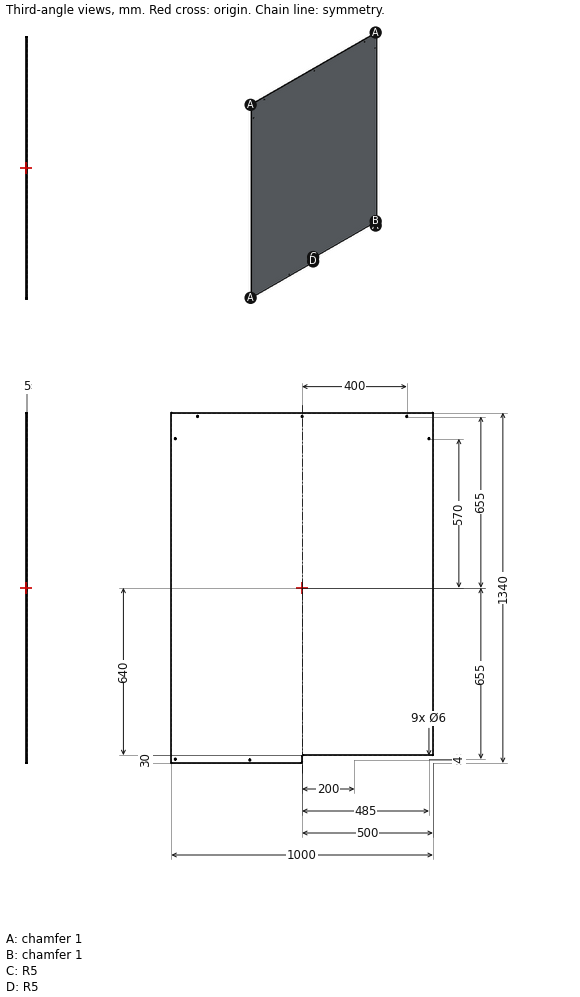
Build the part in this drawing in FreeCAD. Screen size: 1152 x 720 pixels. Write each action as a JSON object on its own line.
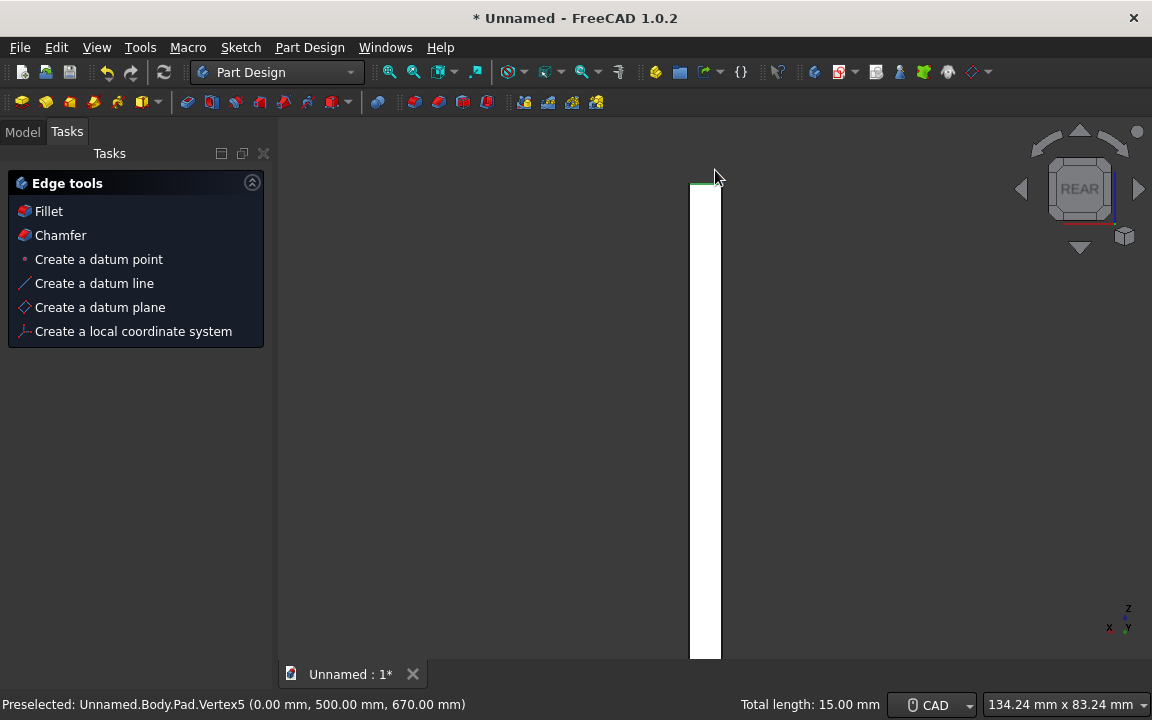
{"action": "left_click", "coordinate": [390, 72]}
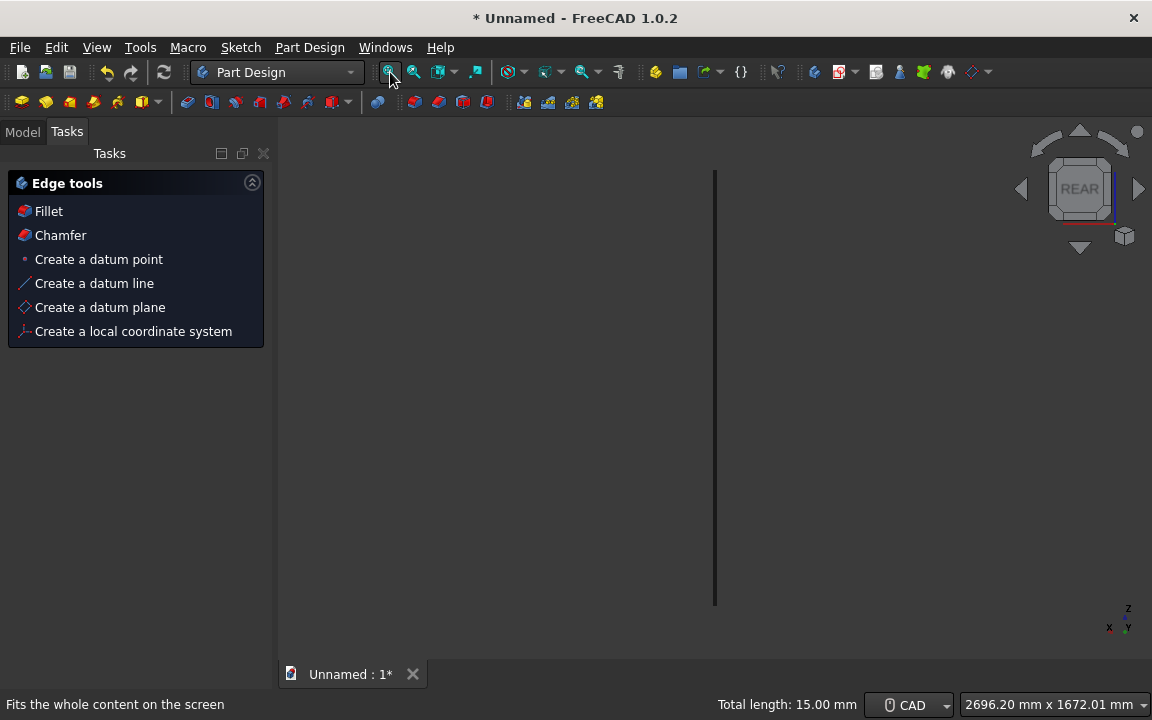
{"action": "key", "text": "6"}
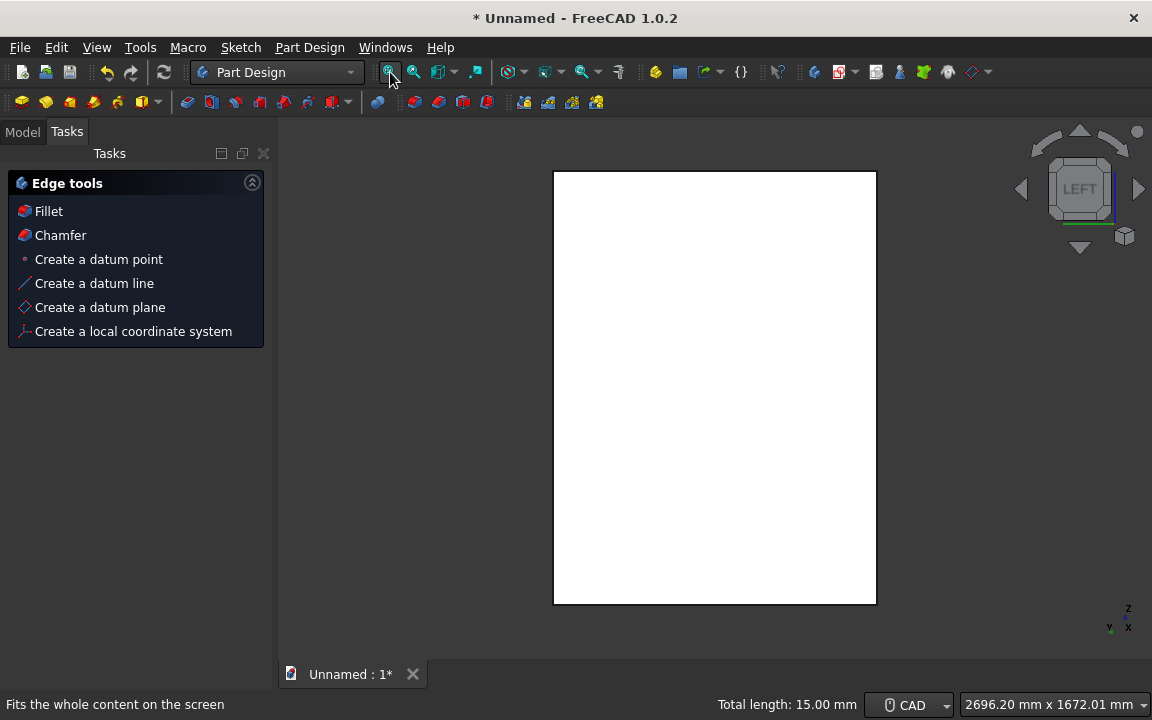
{"action": "scroll", "coordinate": [877, 170], "scroll_direction": "up", "scroll_amount": 15}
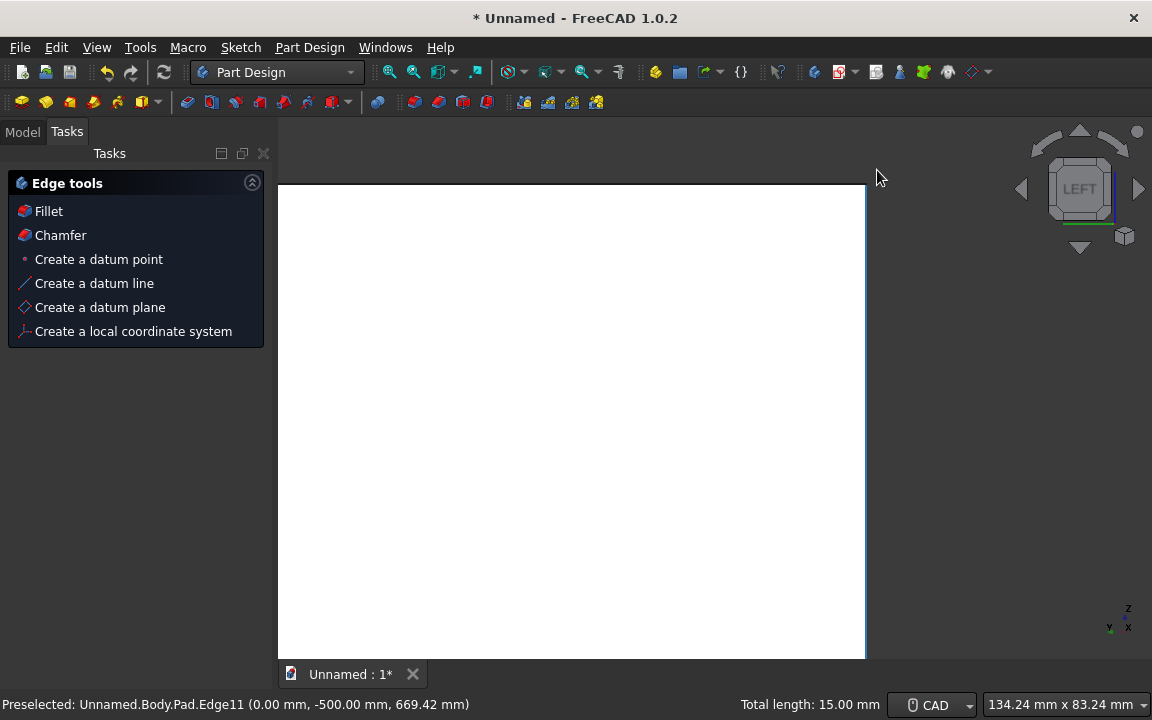
{"action": "left_click", "coordinate": [390, 72]}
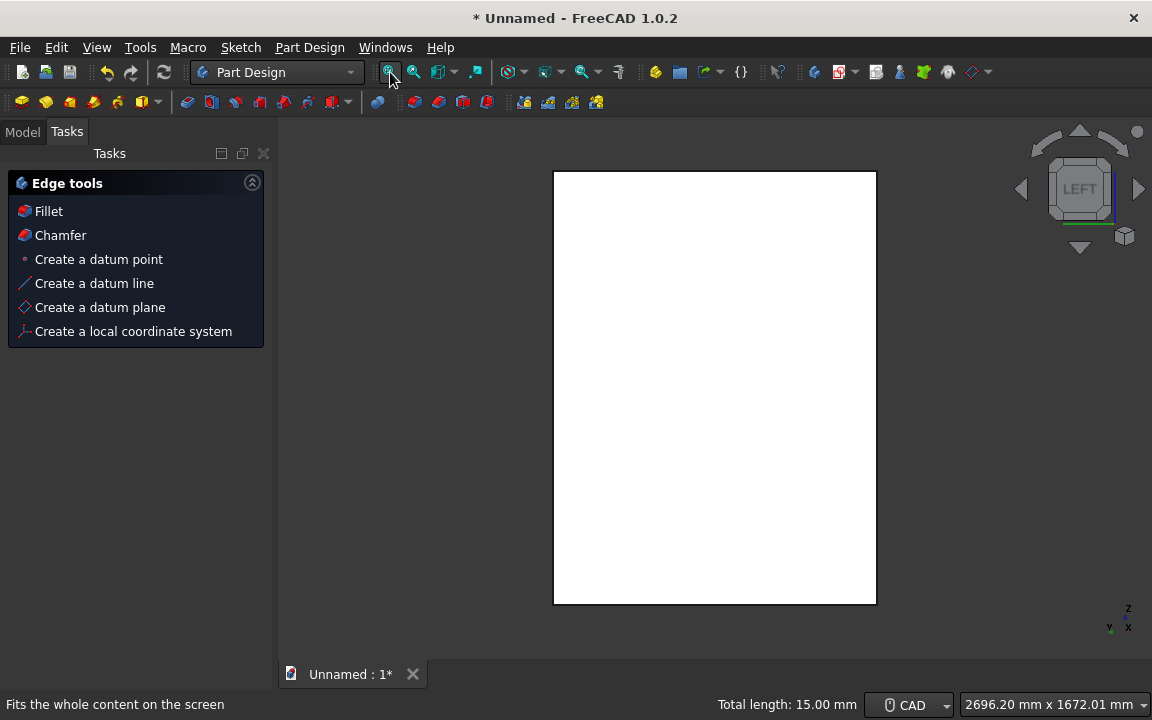
{"action": "key", "text": "v 3"}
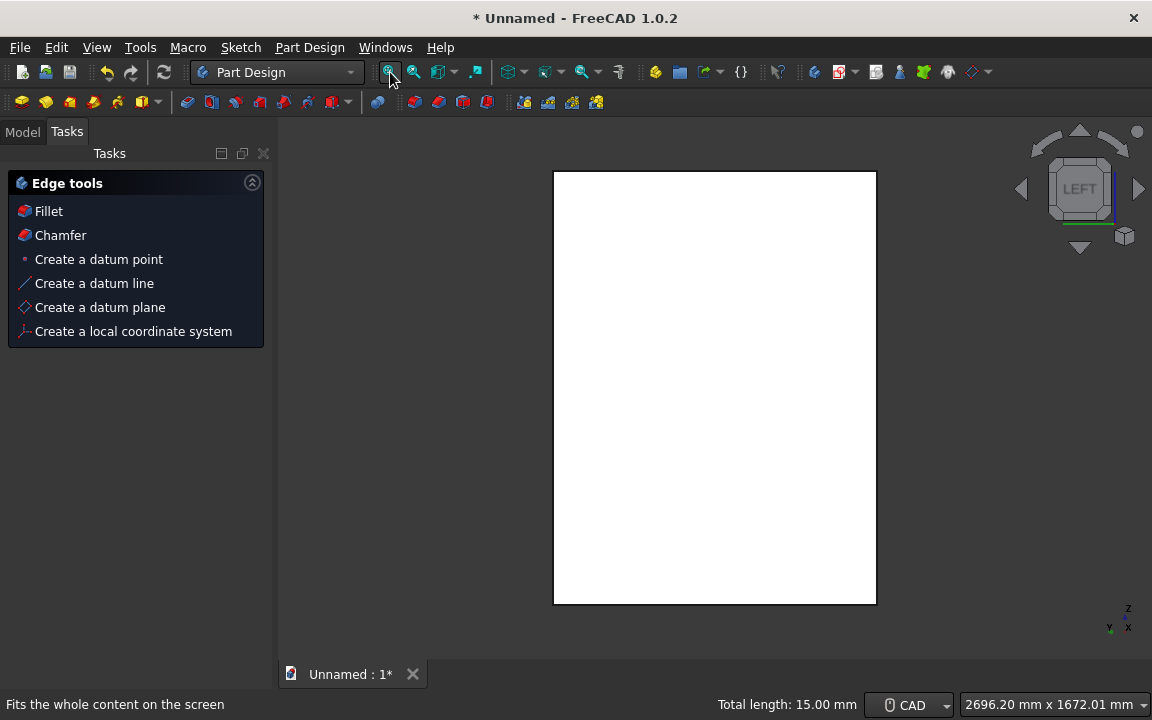
{"action": "key", "text": "0"}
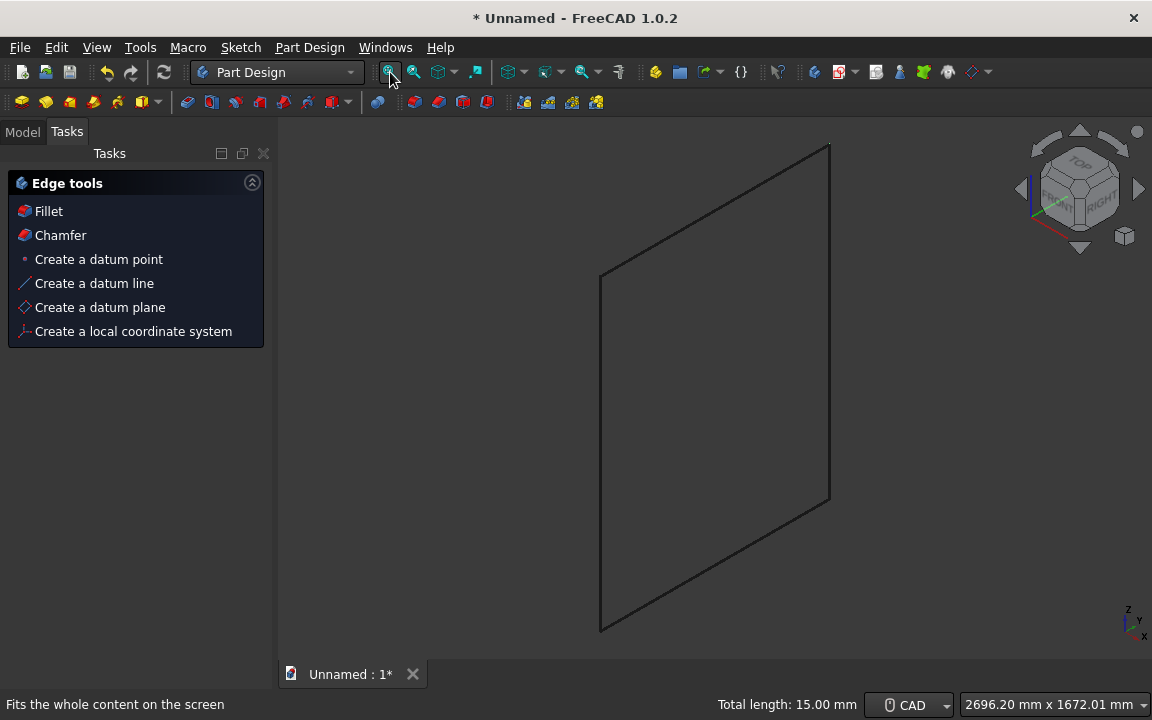
{"action": "scroll", "coordinate": [600, 276], "scroll_direction": "up", "scroll_amount": 15}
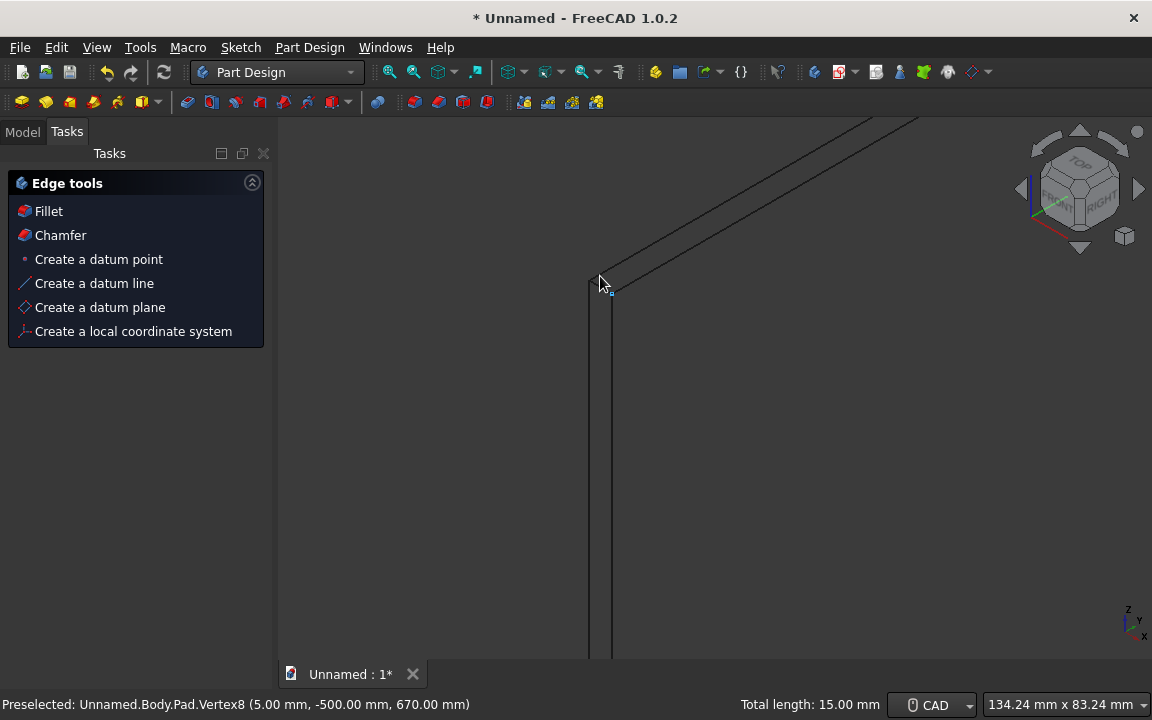
{"action": "left_click", "coordinate": [601, 286], "text": "ctrl"}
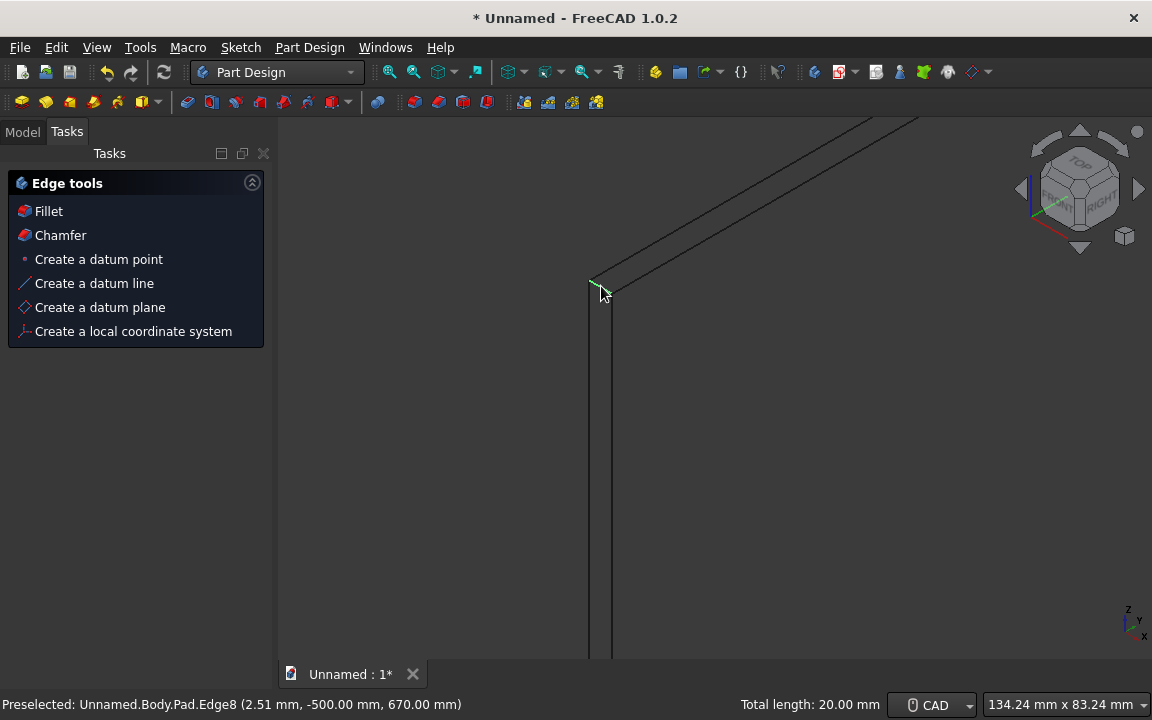
{"action": "key", "text": "v 1"}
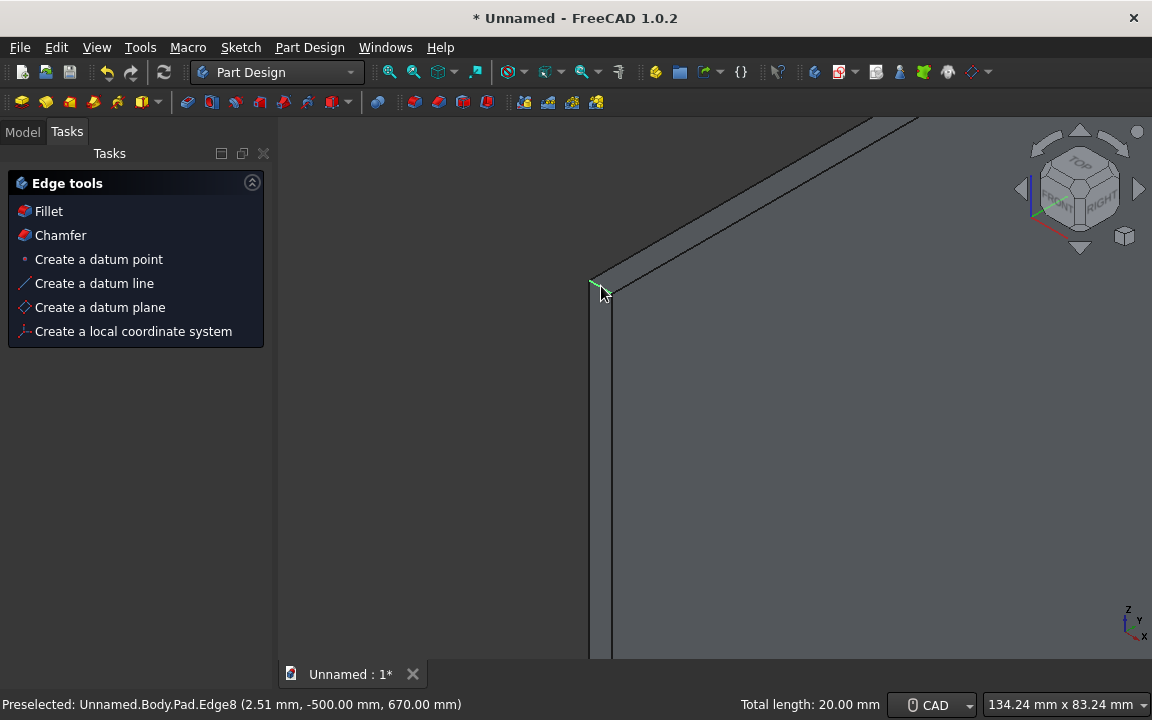
{"action": "left_click", "coordinate": [440, 102]}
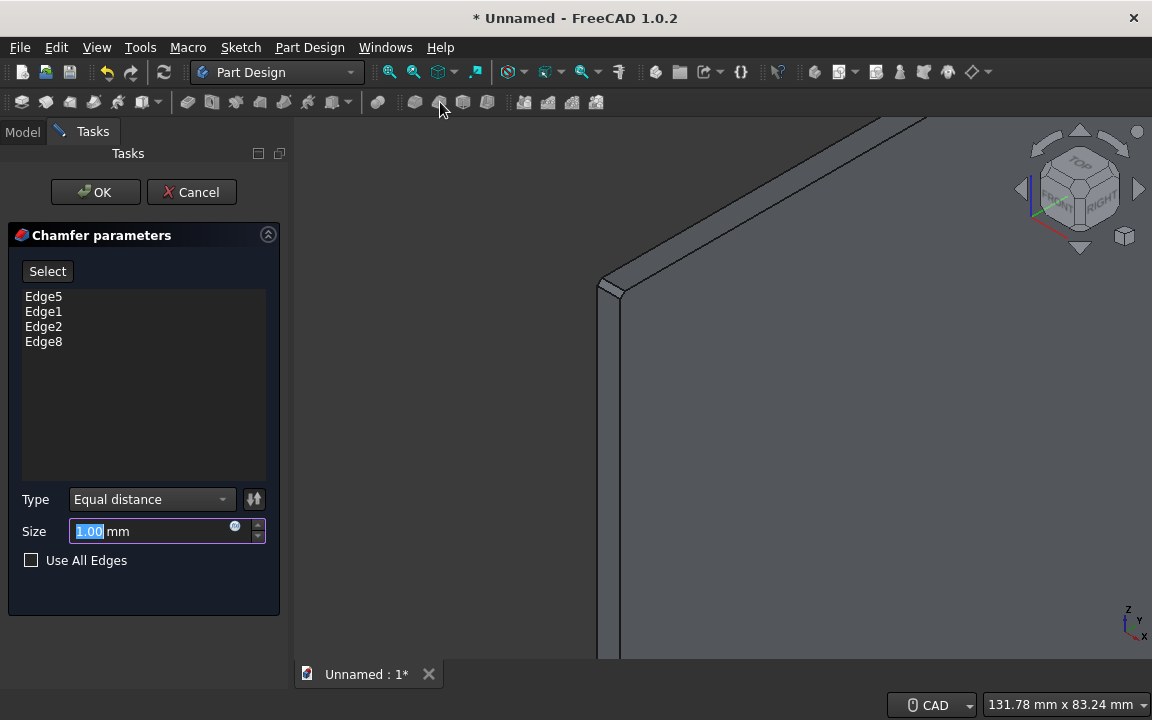
{"action": "type", "text": "1"}
{"action": "key", "text": "Tab"}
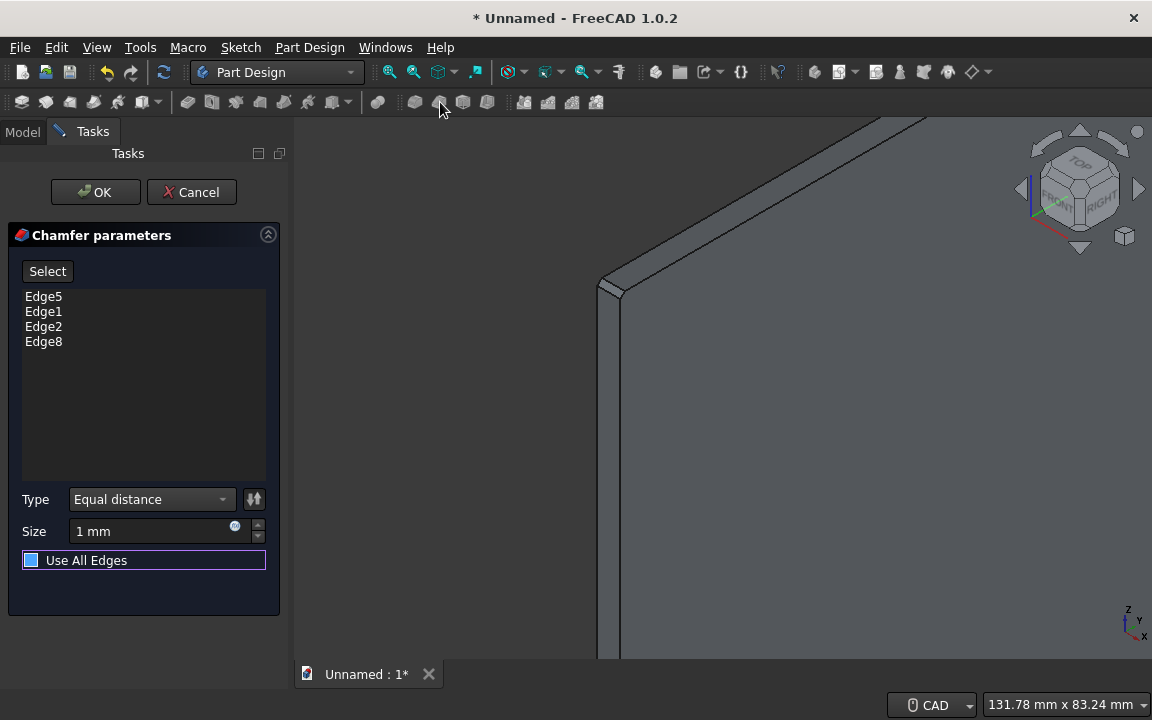
{"action": "left_click", "coordinate": [96, 192]}